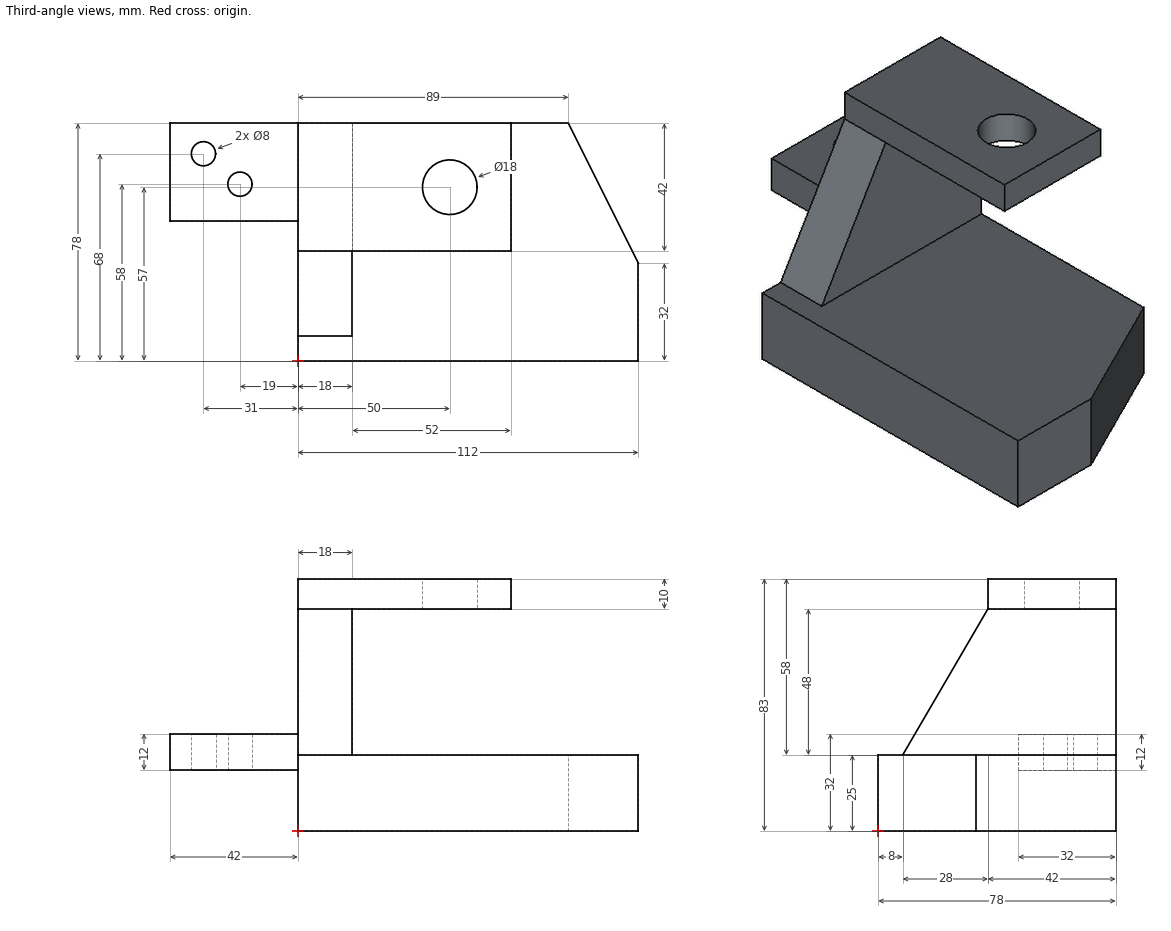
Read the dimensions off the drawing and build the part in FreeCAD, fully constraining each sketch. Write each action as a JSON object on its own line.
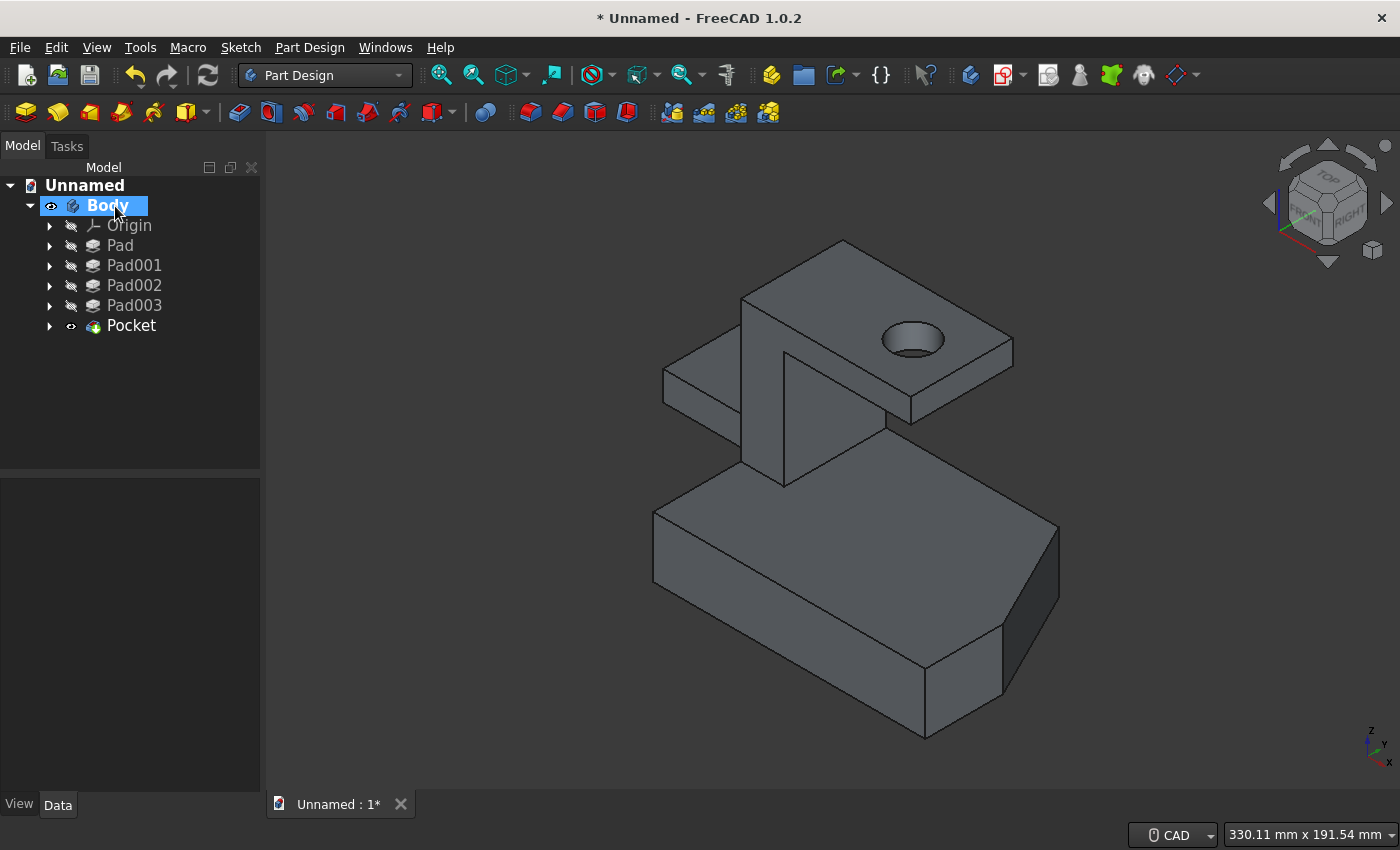
{"action": "key", "text": "2"}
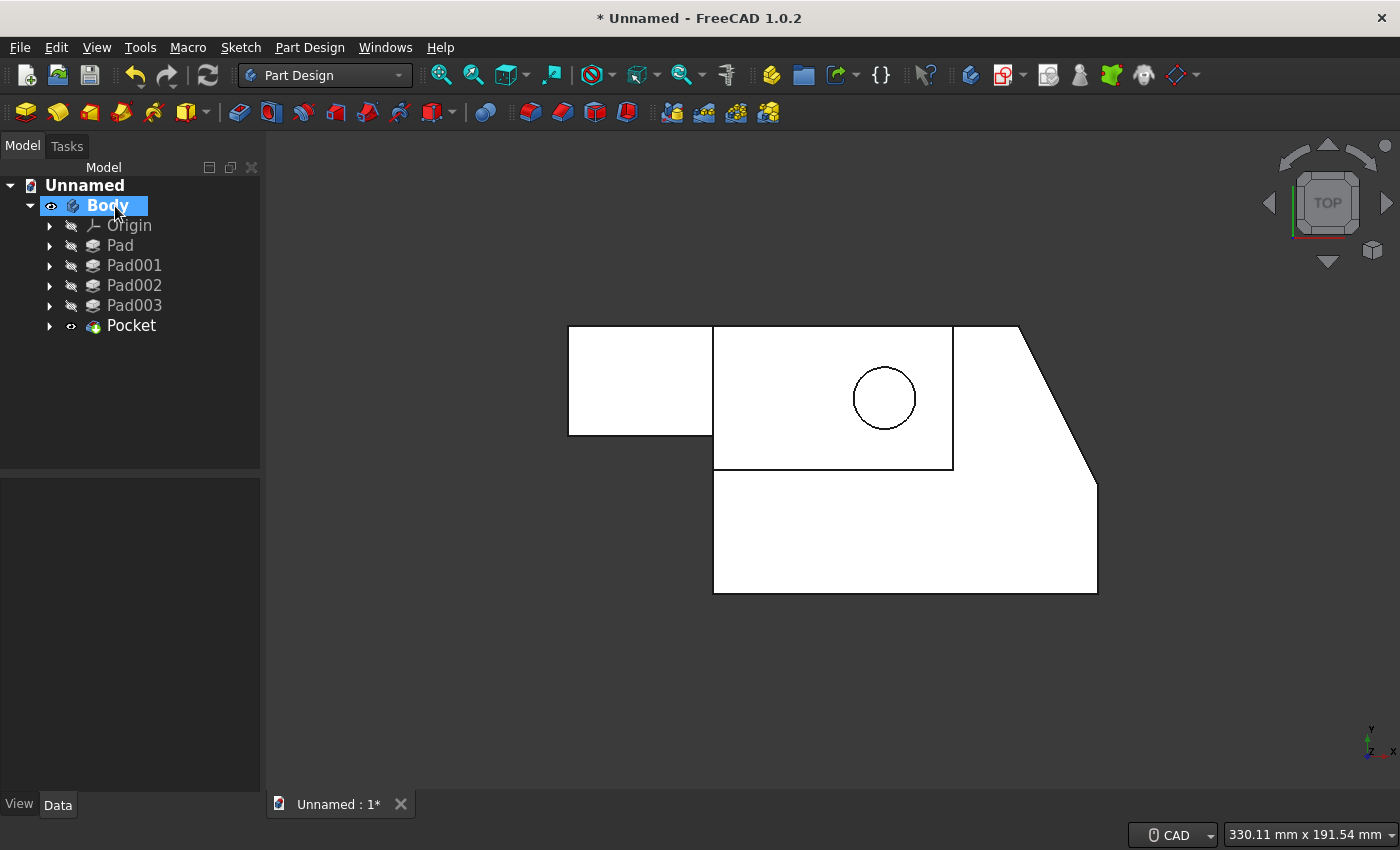
{"action": "left_click", "coordinate": [641, 380]}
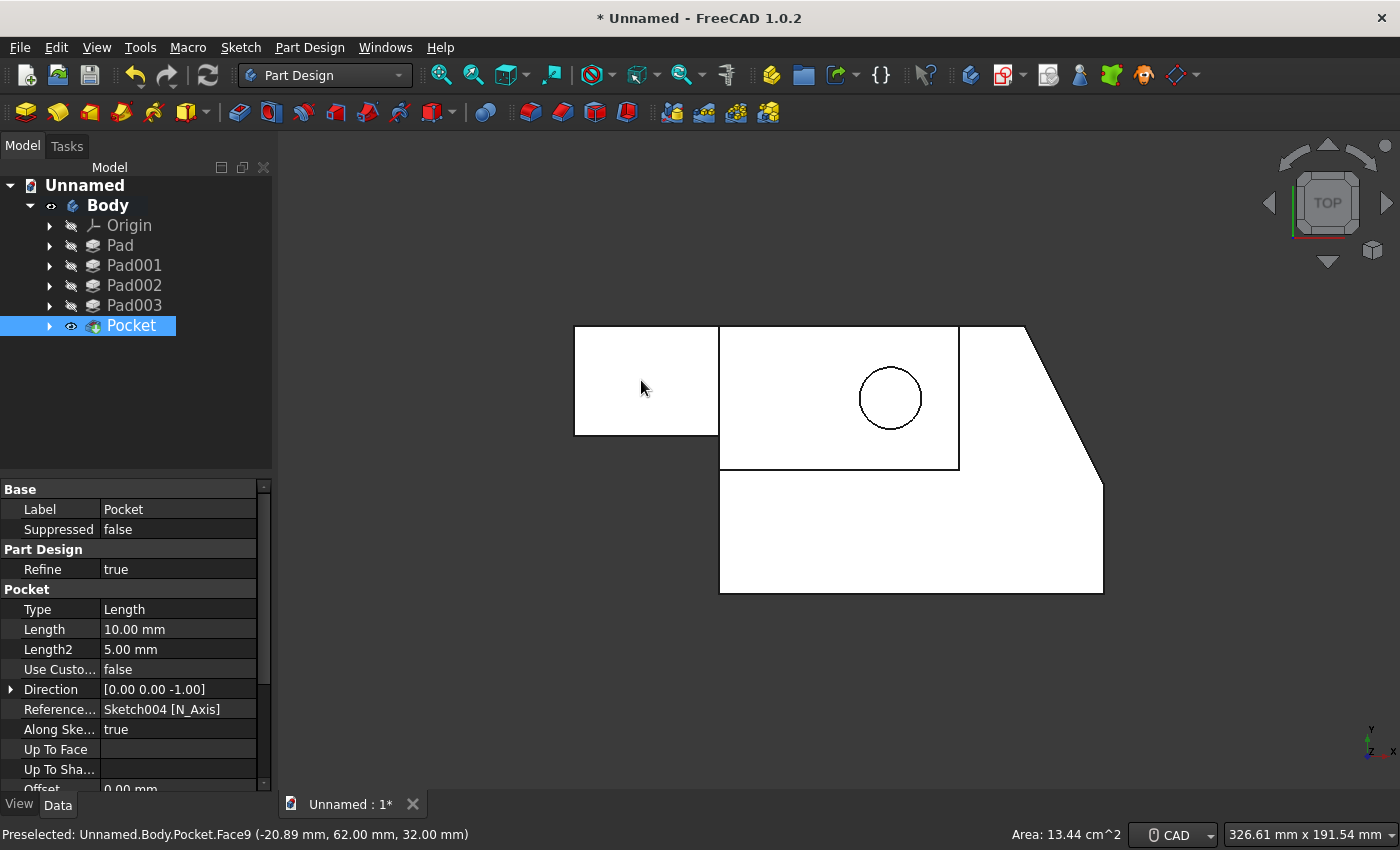
{"action": "left_click", "coordinate": [1004, 76]}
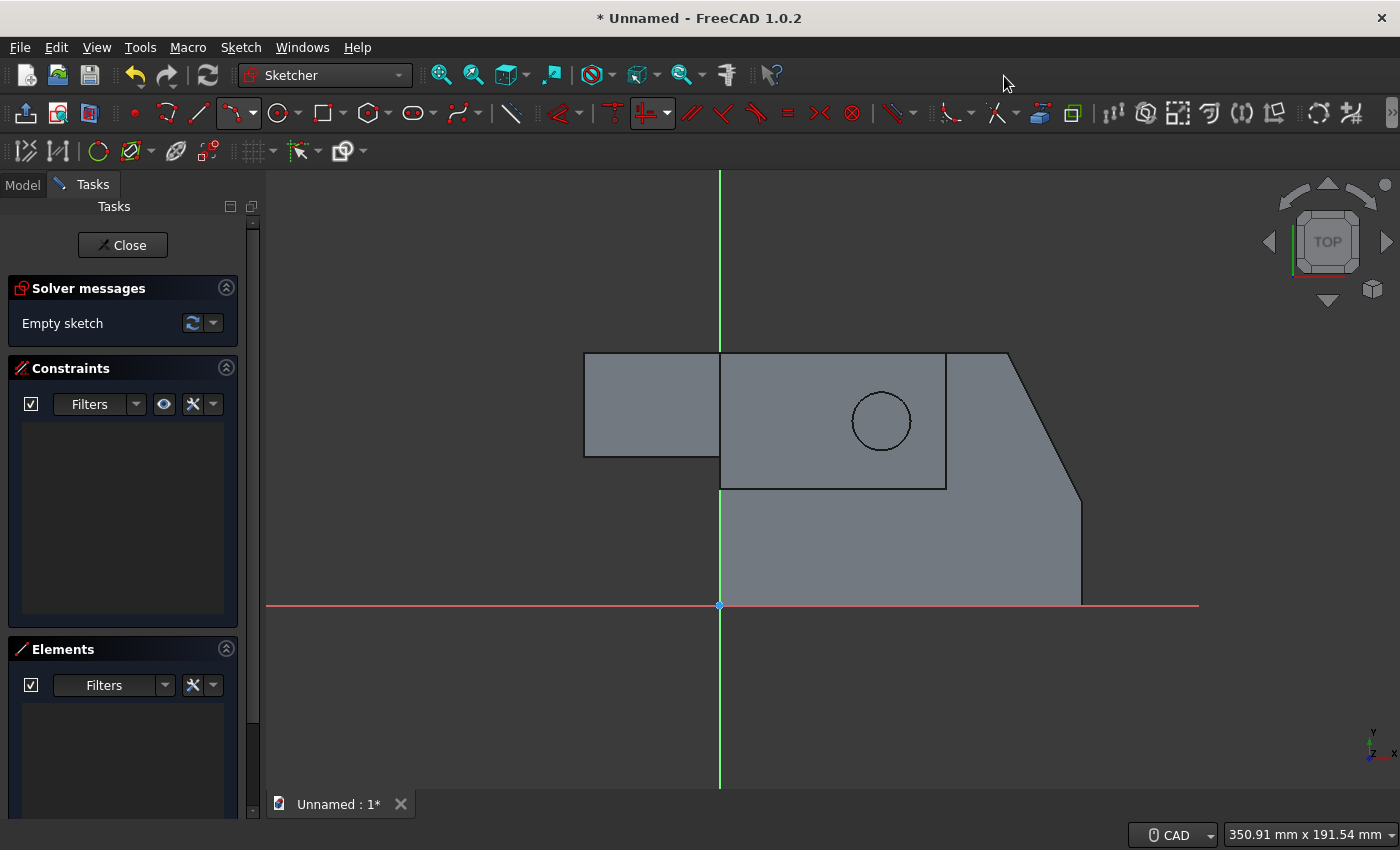
{"action": "left_click", "coordinate": [90, 114]}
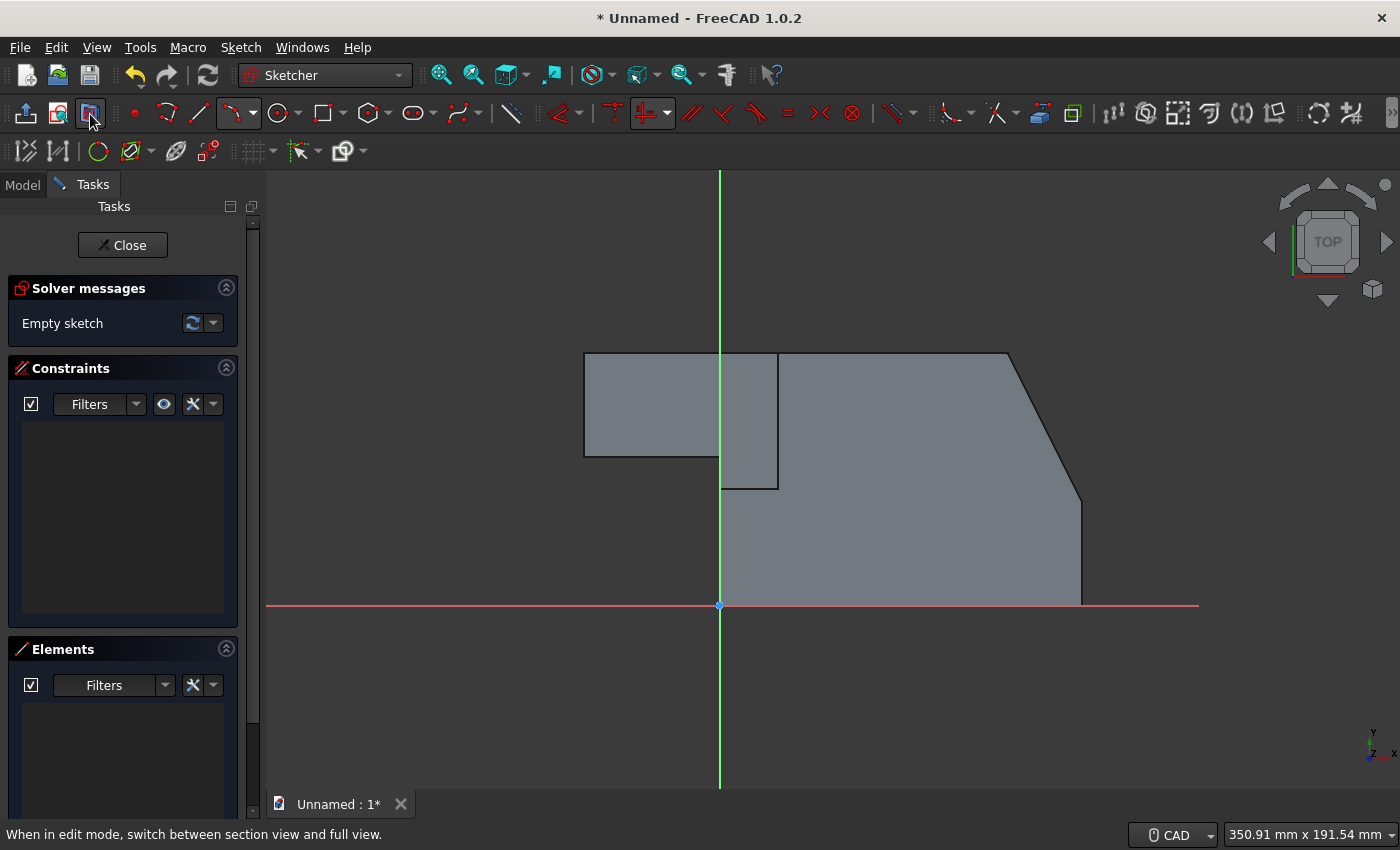
{"action": "scroll", "coordinate": [619, 390], "scroll_direction": "up", "scroll_amount": 10}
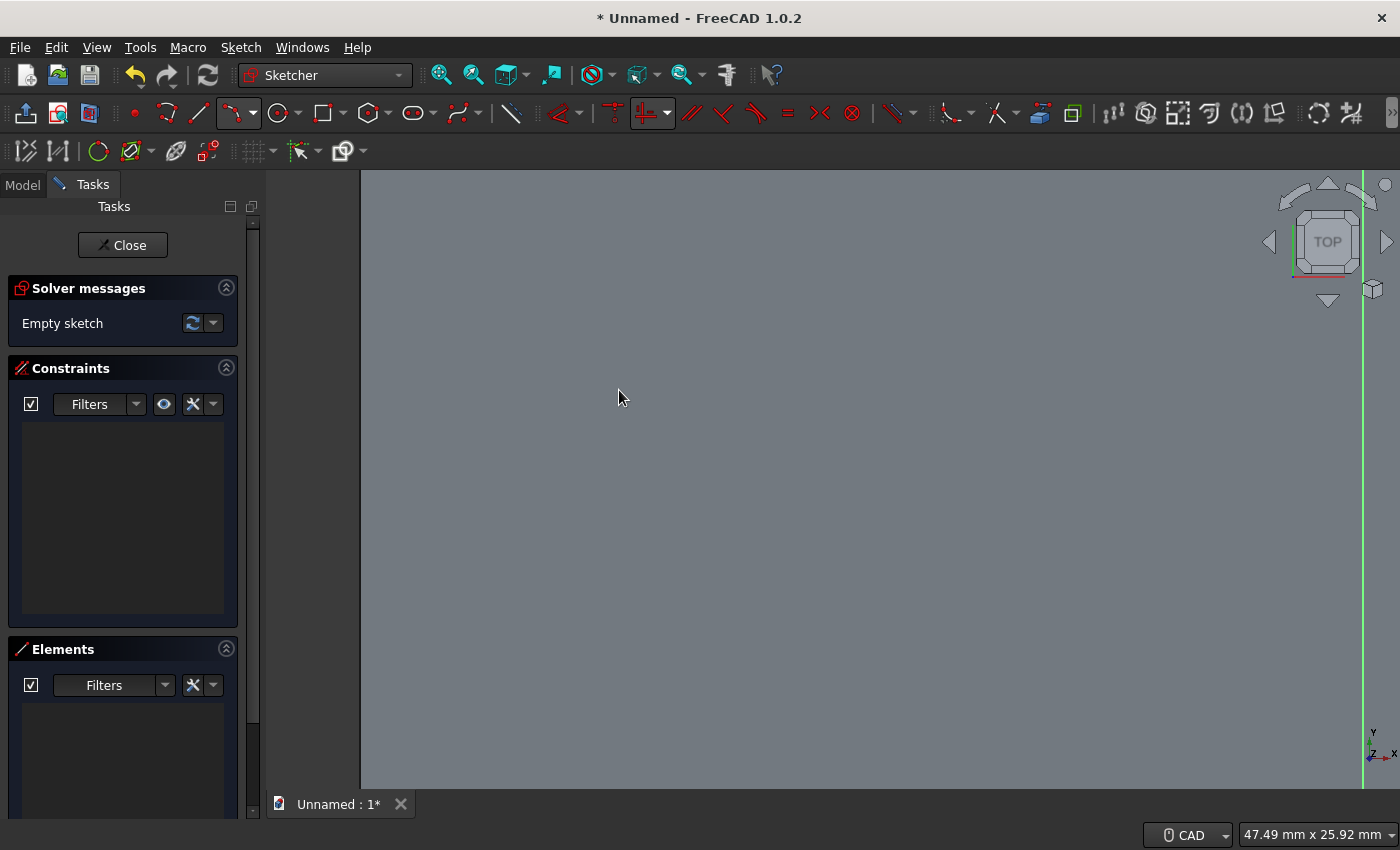
{"action": "key", "text": "g c"}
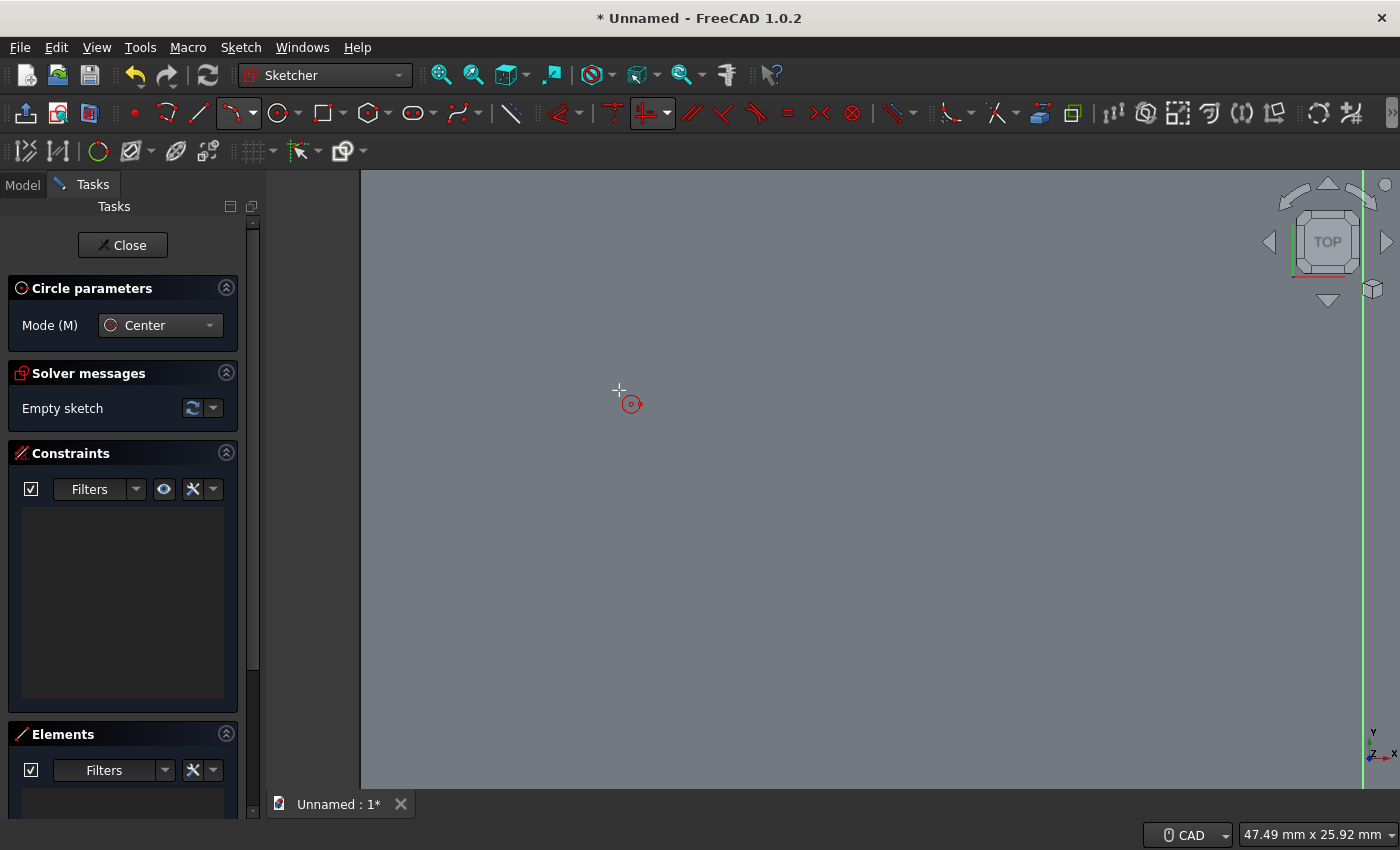
{"action": "left_click", "coordinate": [622, 357]}
{"action": "mouse_move", "coordinate": [690, 289]}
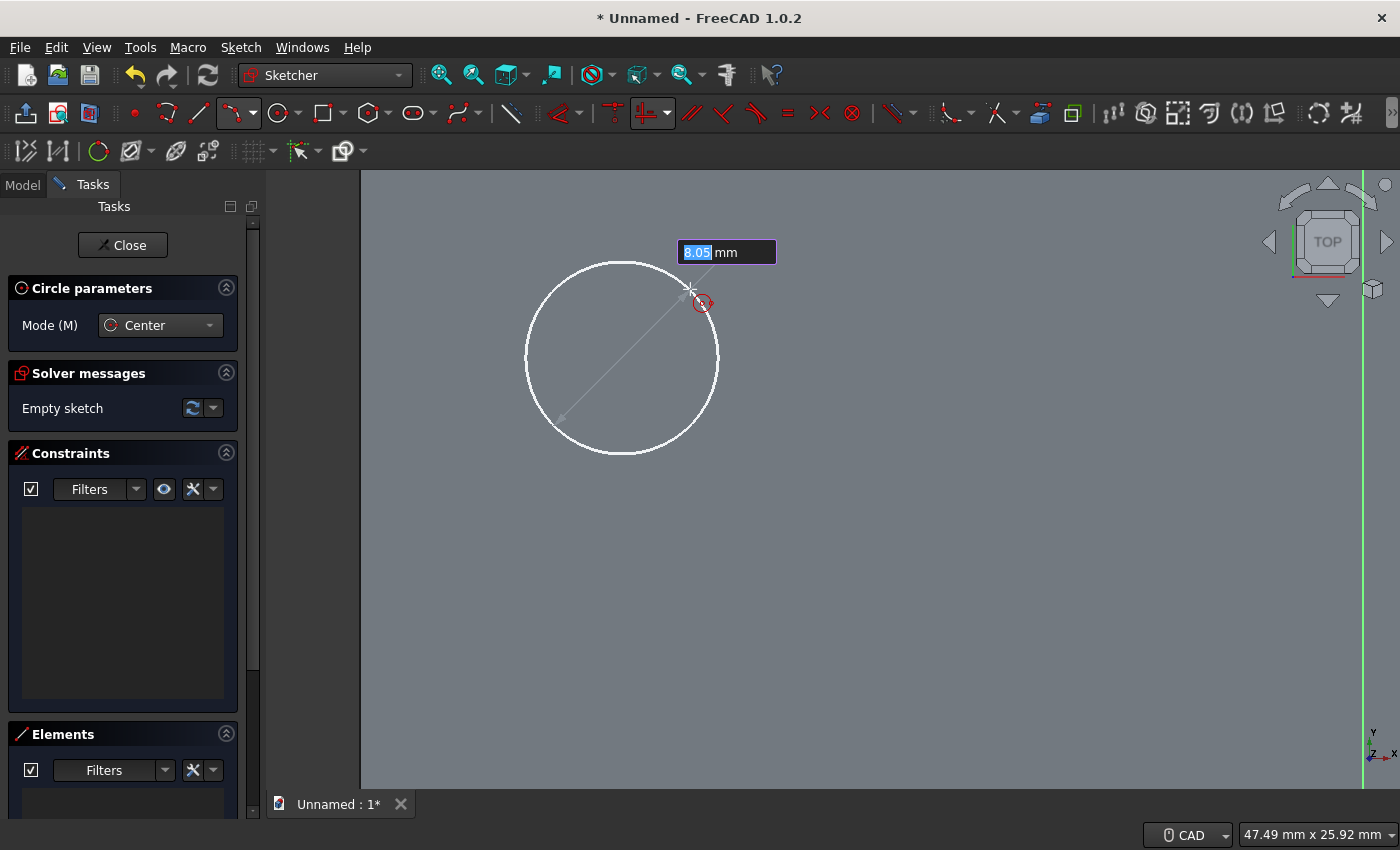
{"action": "type", "text": "8"}
{"action": "key", "text": "Return"}